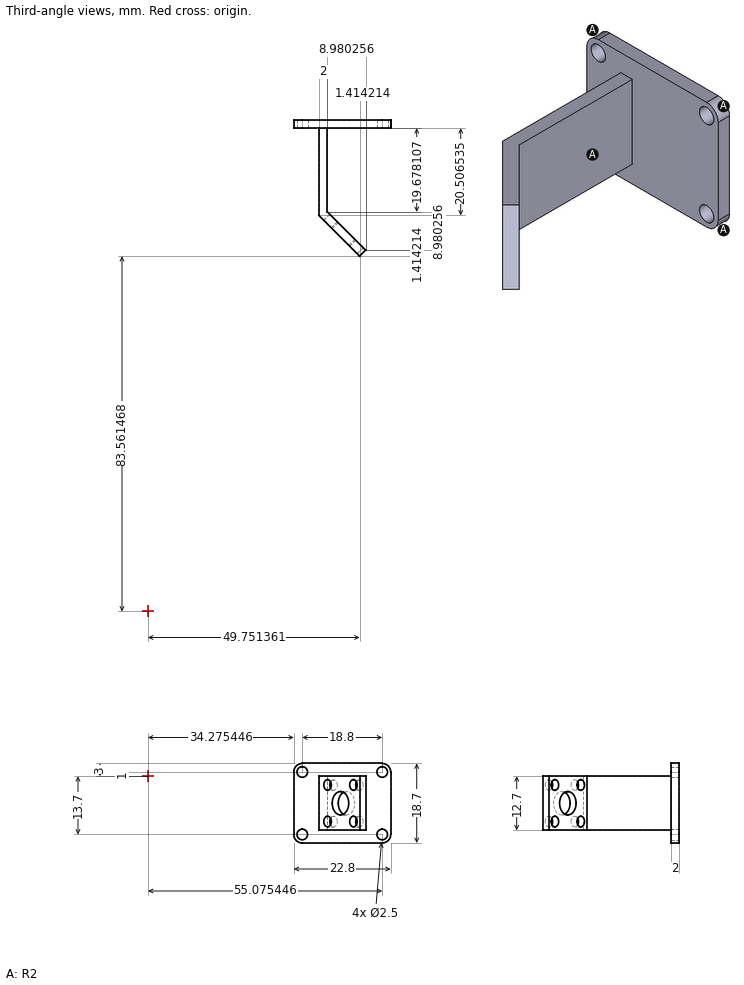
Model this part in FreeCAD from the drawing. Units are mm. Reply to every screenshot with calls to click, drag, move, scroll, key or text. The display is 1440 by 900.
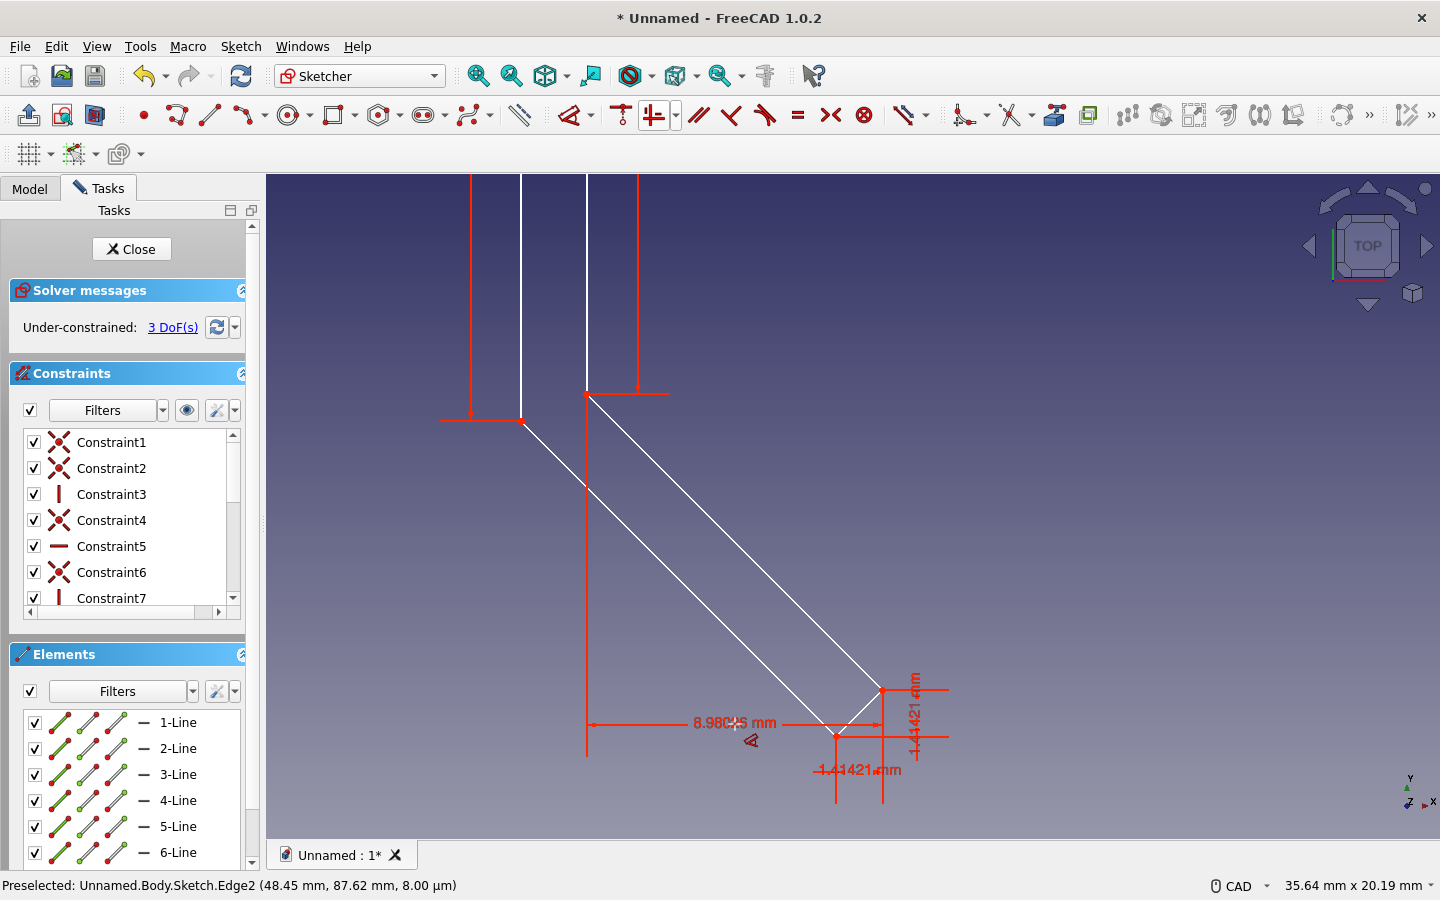
click(794, 601)
click(917, 542)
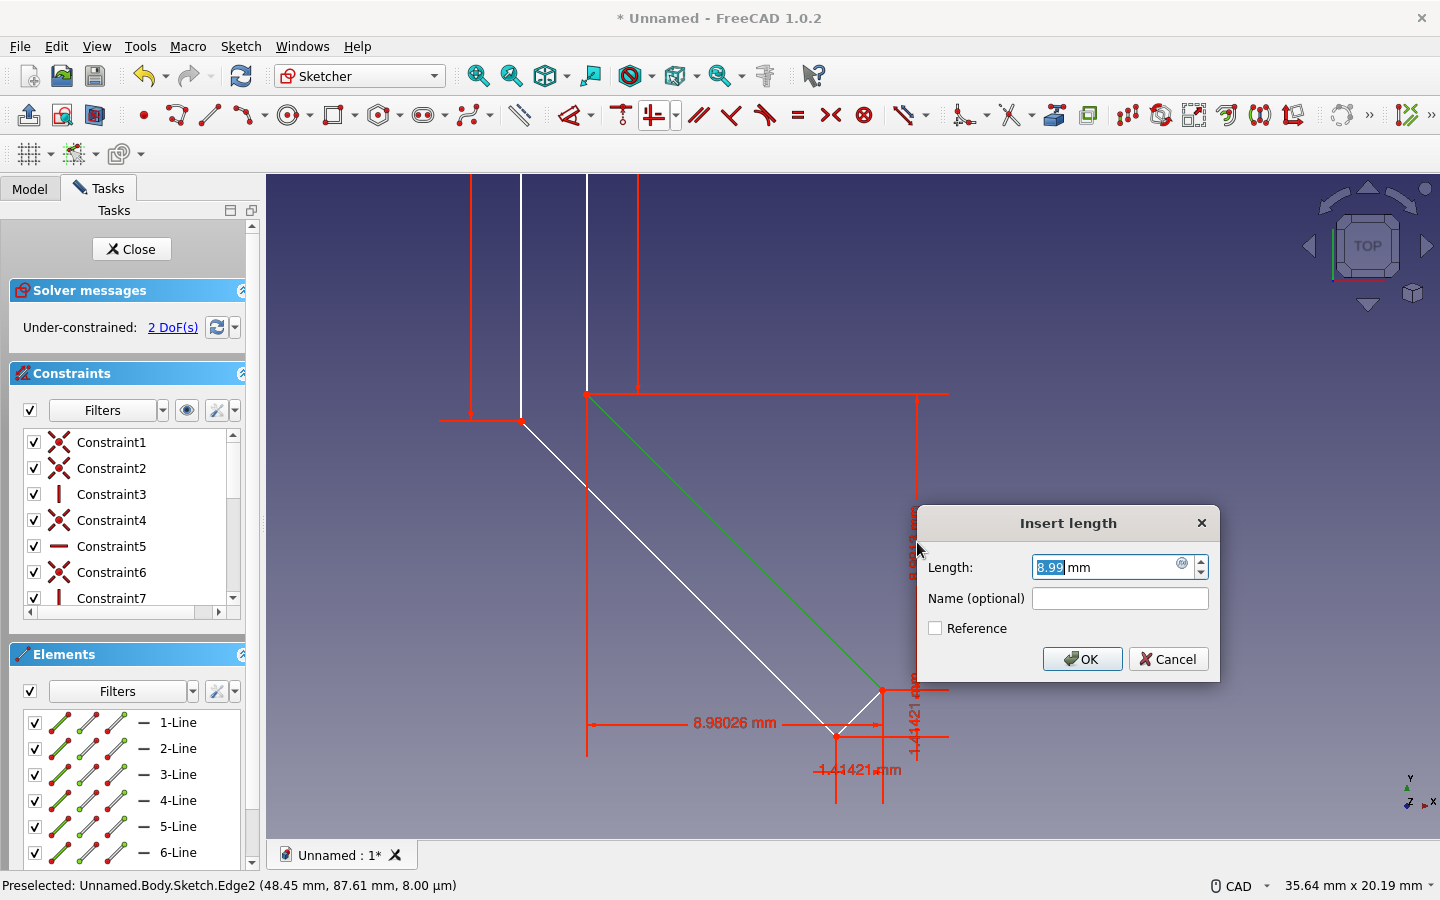
text(8.980256)
key(Return)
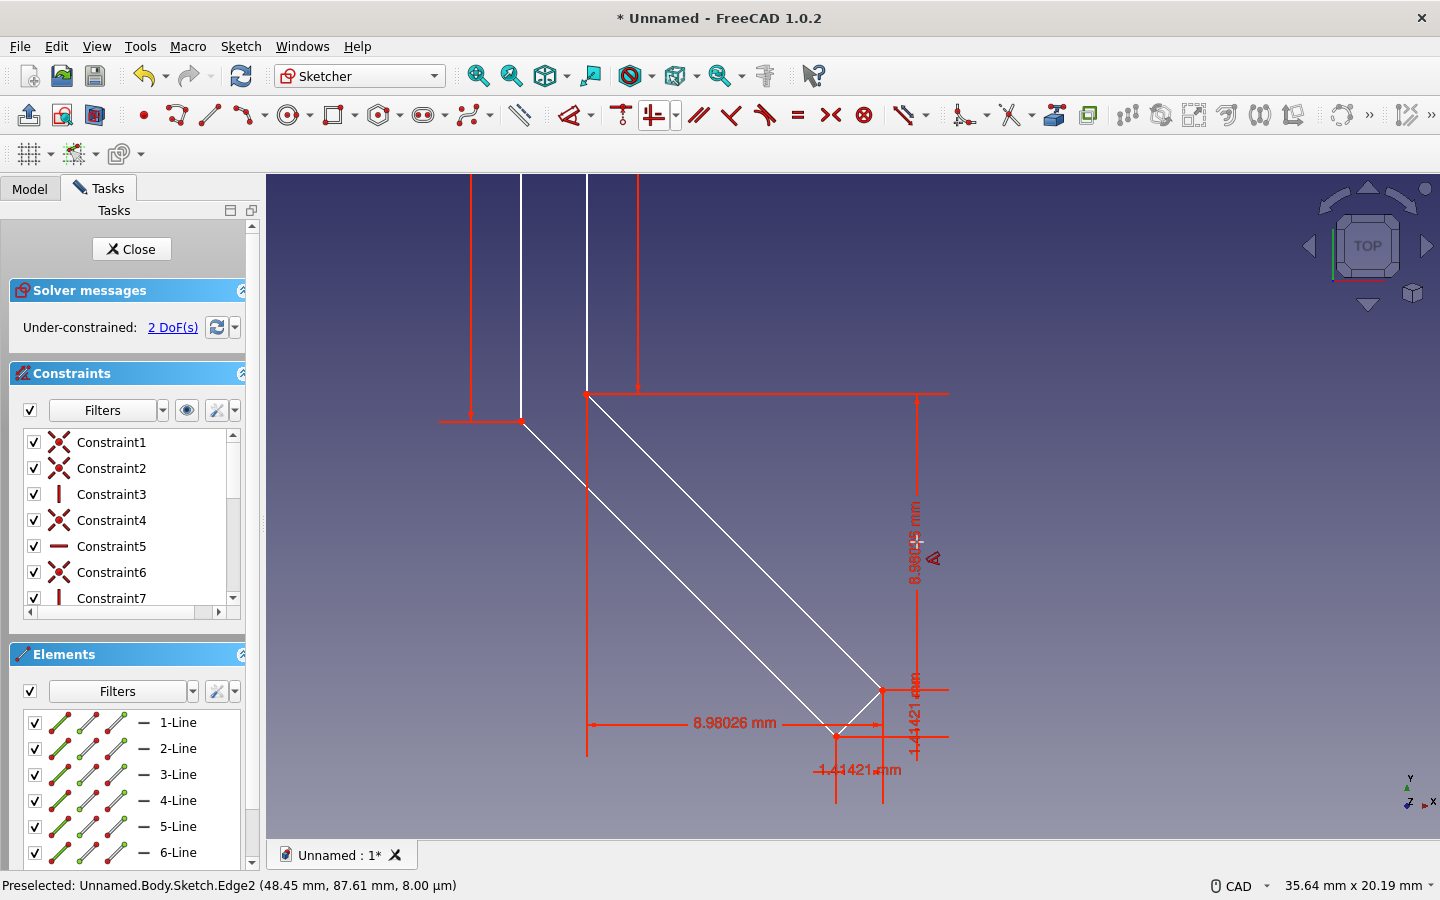
click(836, 737)
click(565, 703)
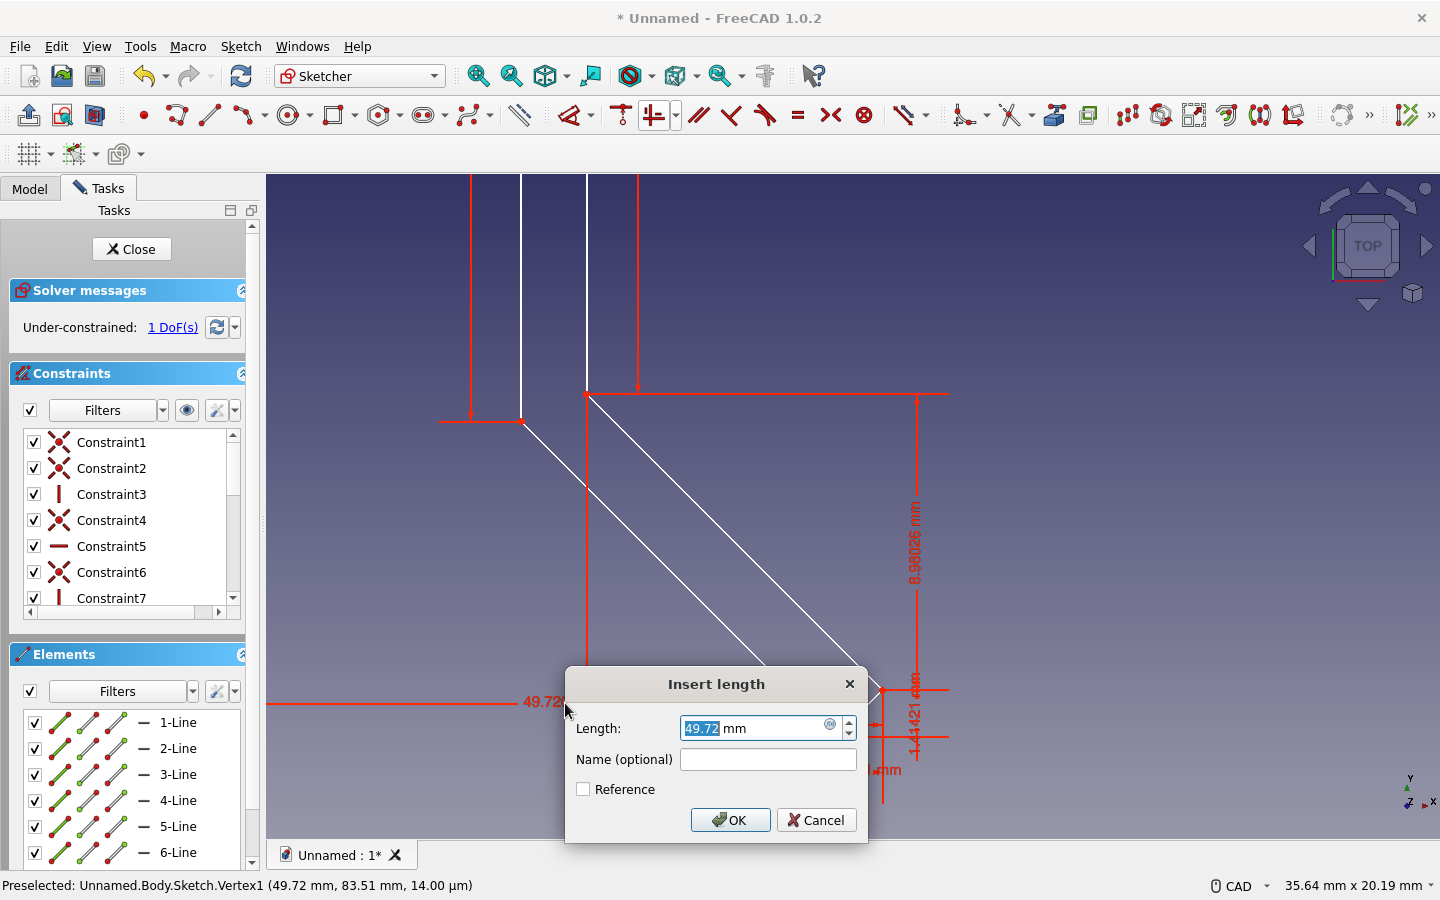
text(49.751361)
key(Return)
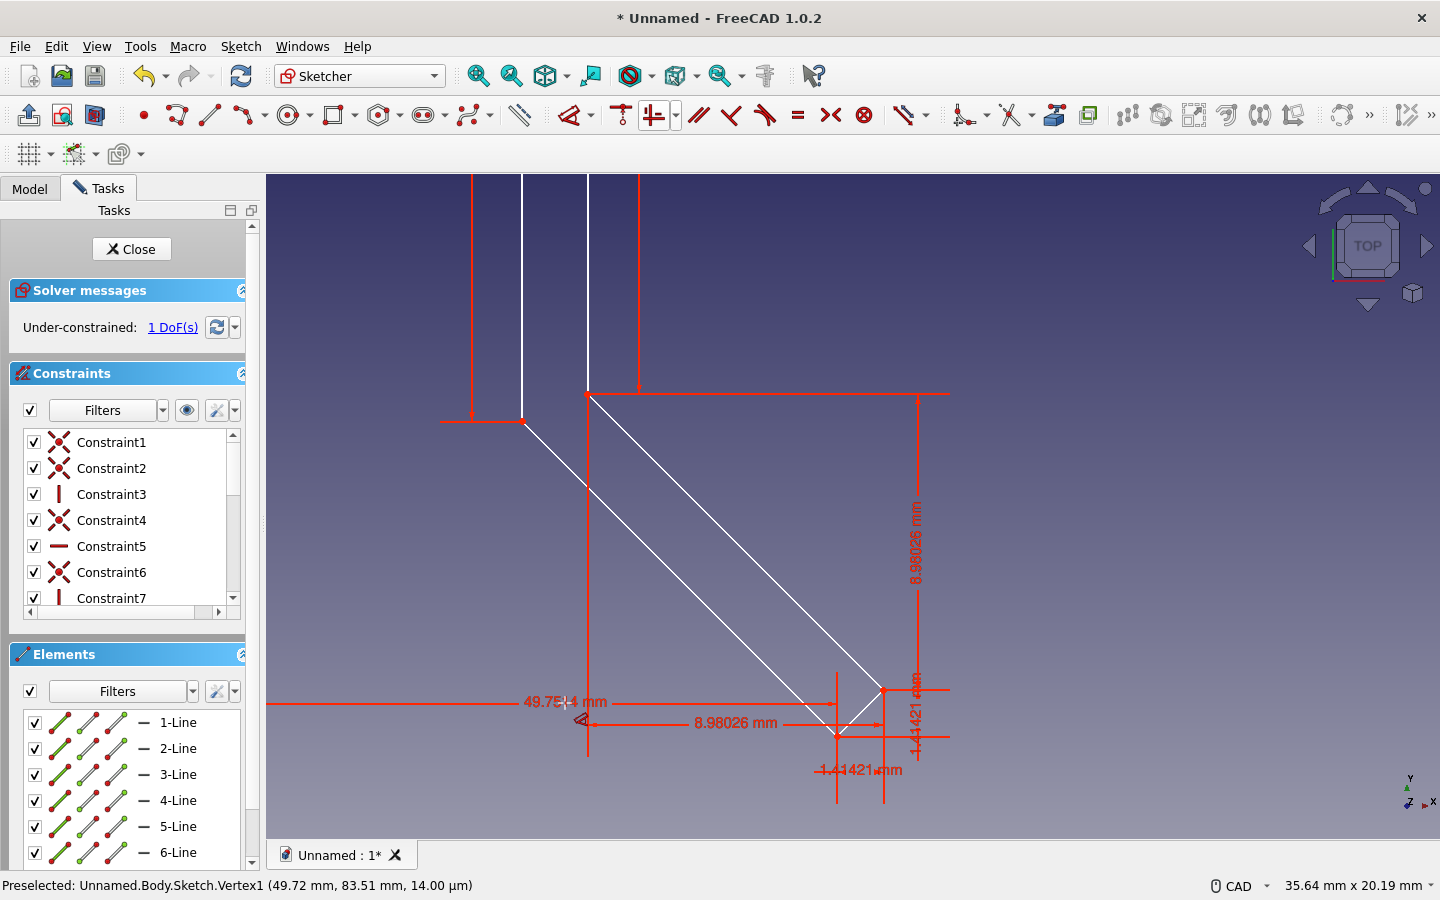
click(837, 737)
click(871, 791)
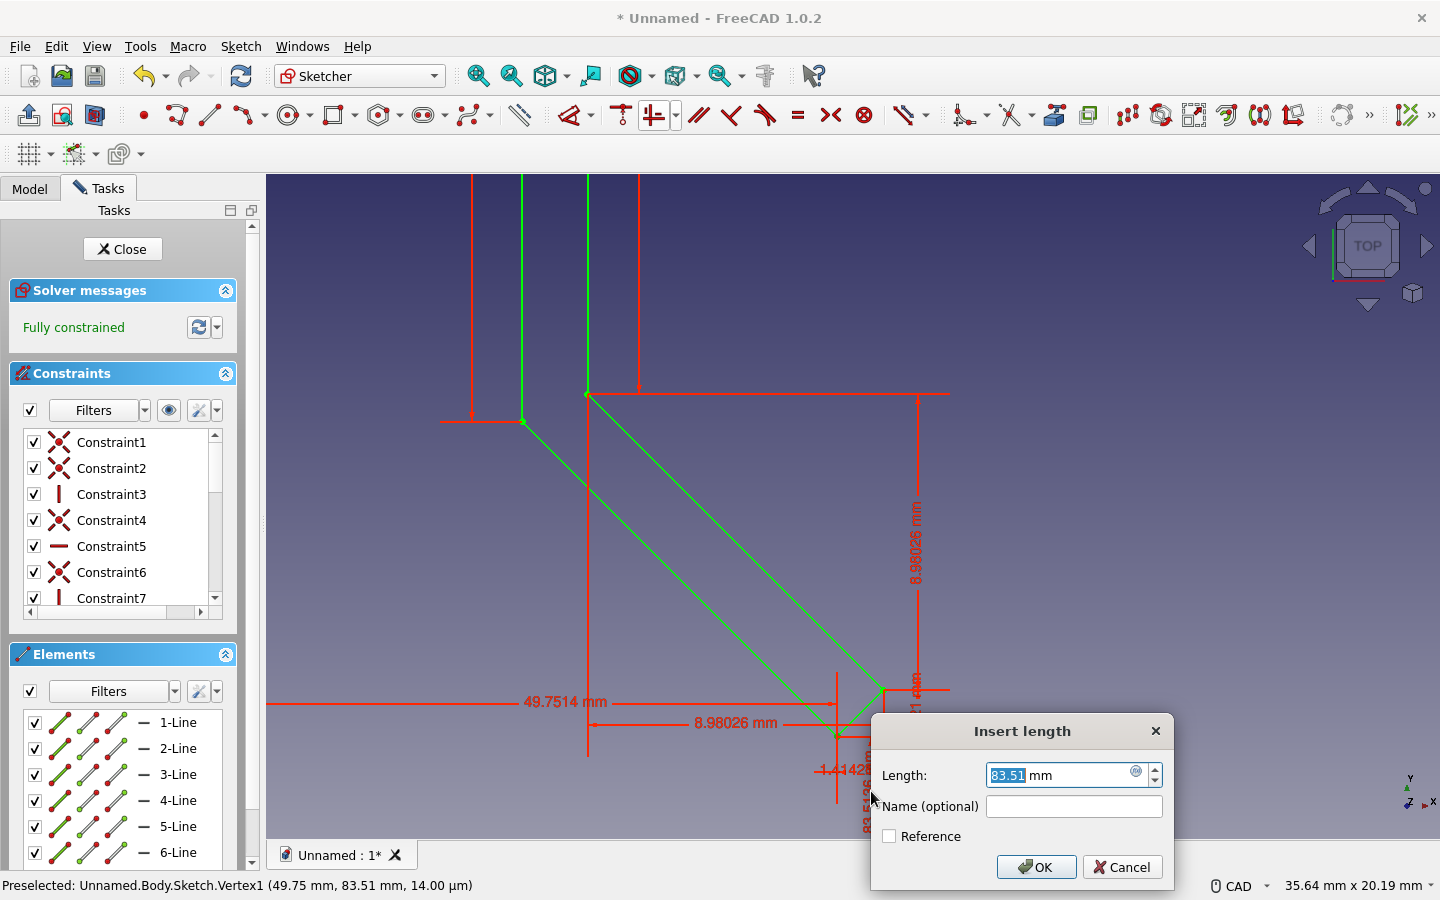
text(83.561468)
key(Return)
key(Escape)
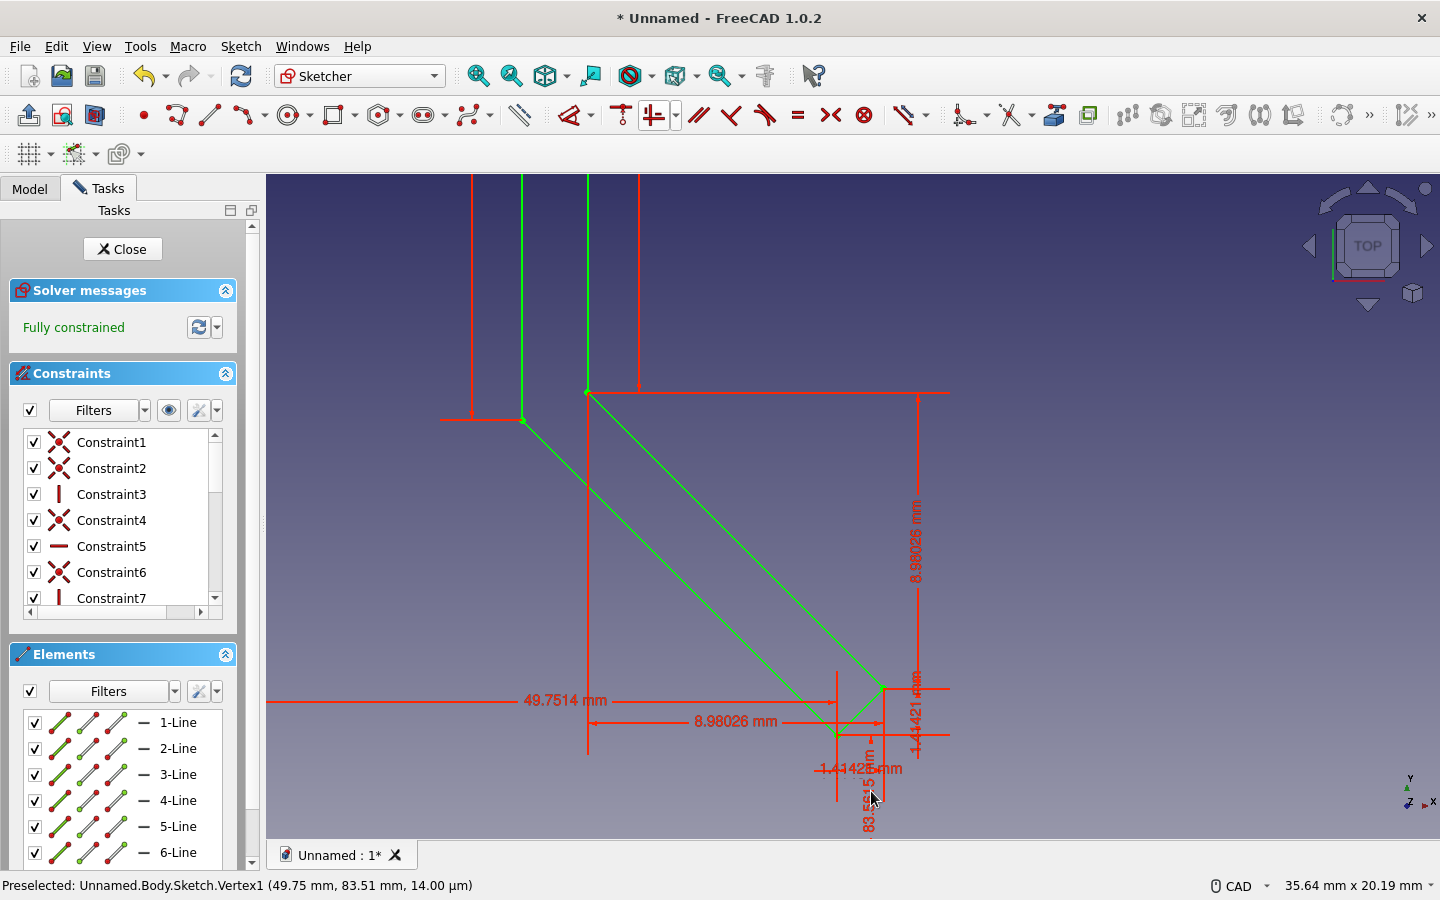
click(123, 249)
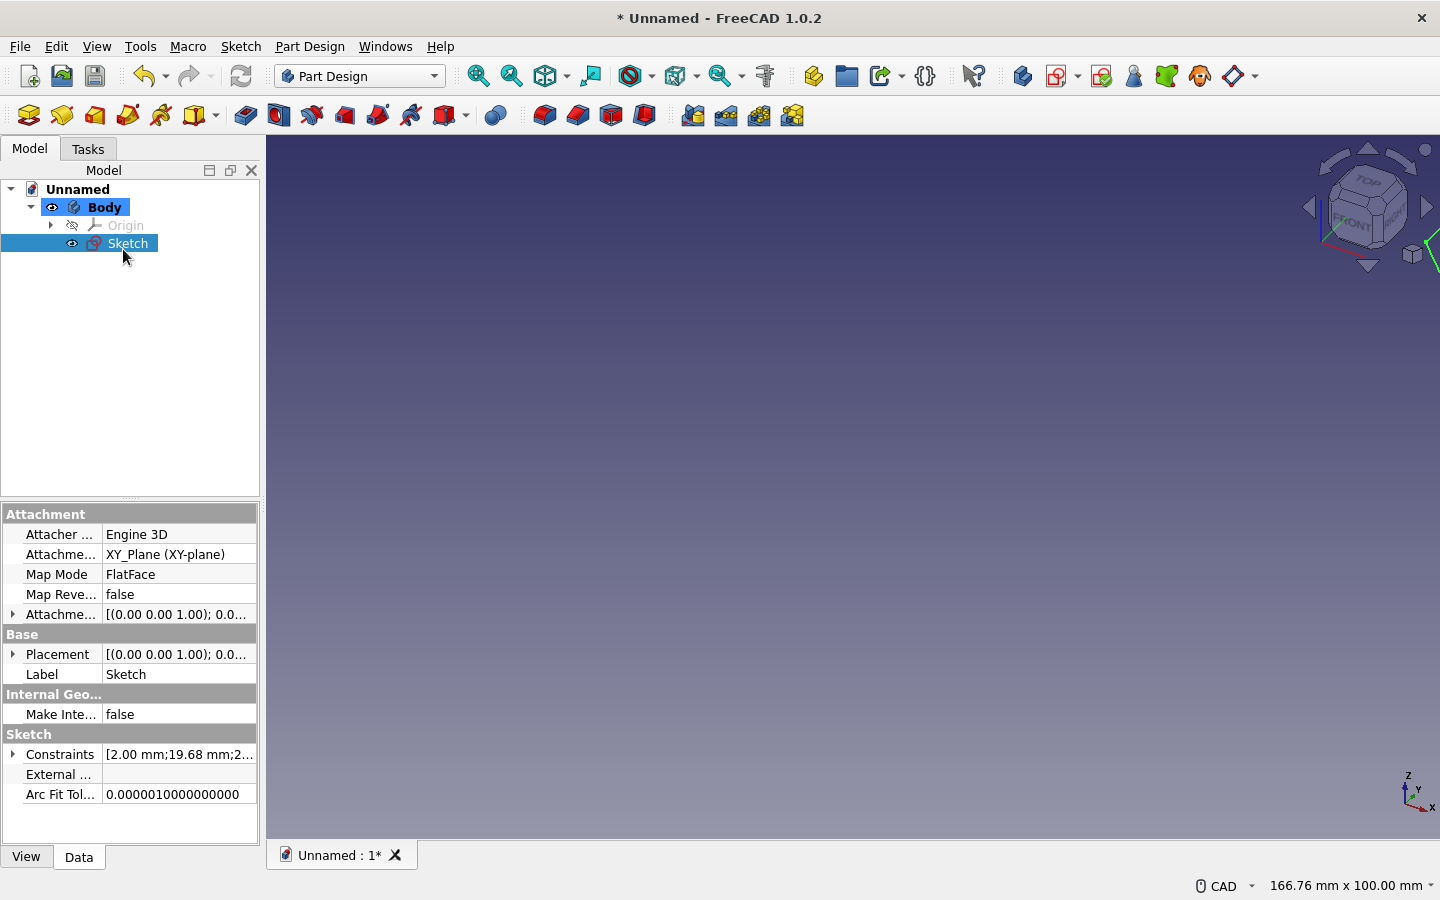
click(29, 116)